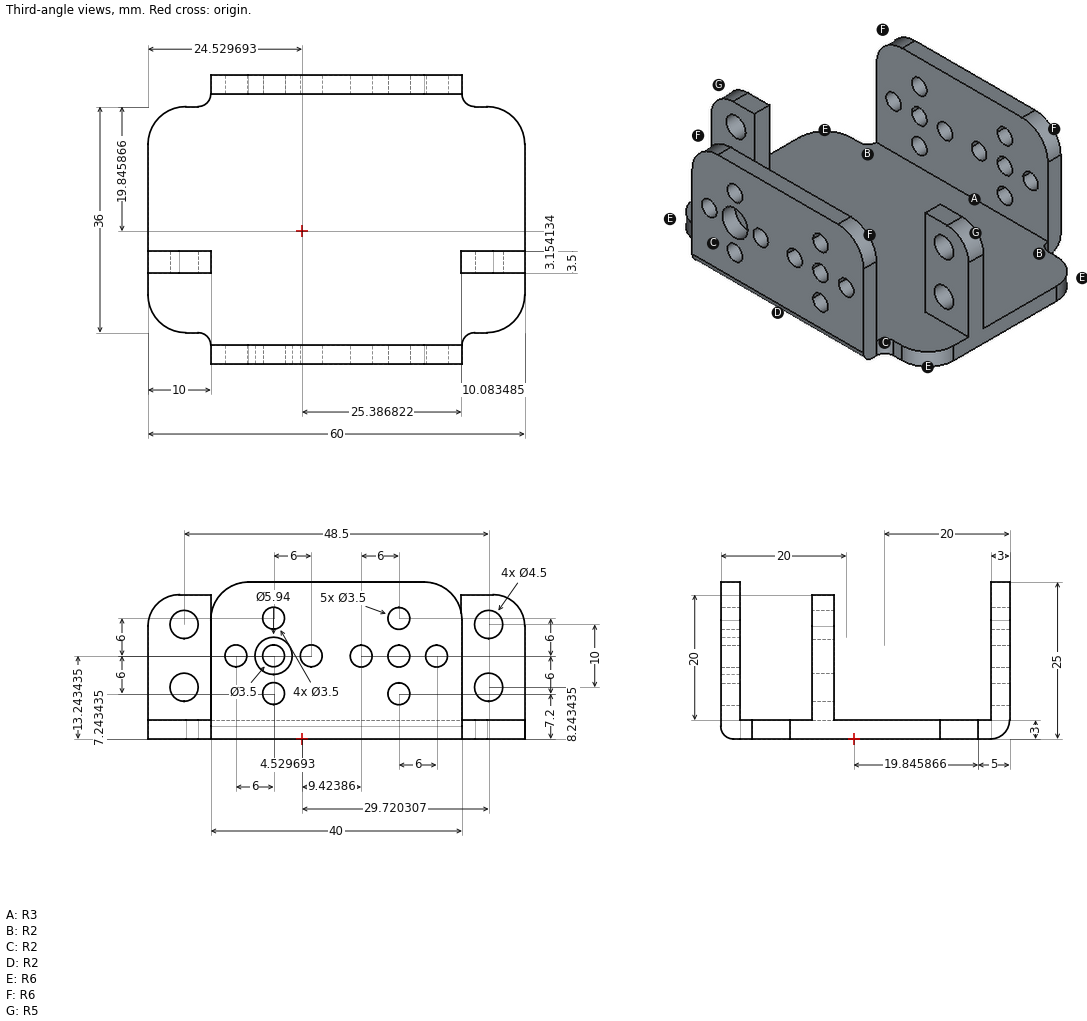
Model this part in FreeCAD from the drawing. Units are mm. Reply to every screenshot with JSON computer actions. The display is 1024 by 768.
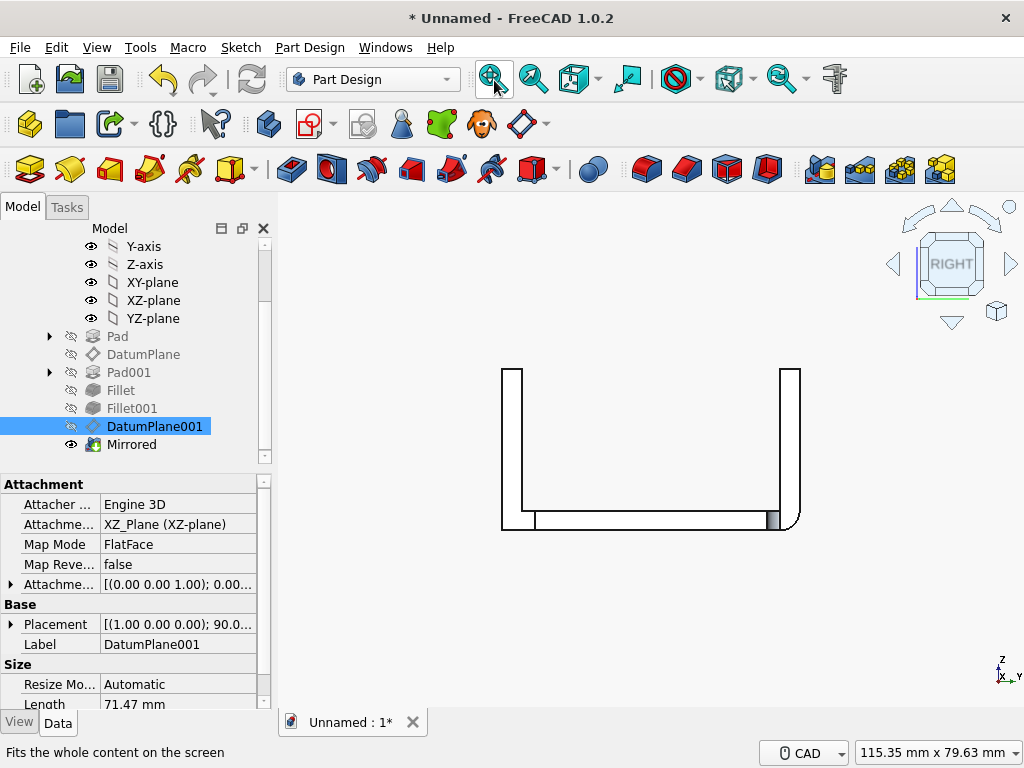
{"action": "key", "text": "5"}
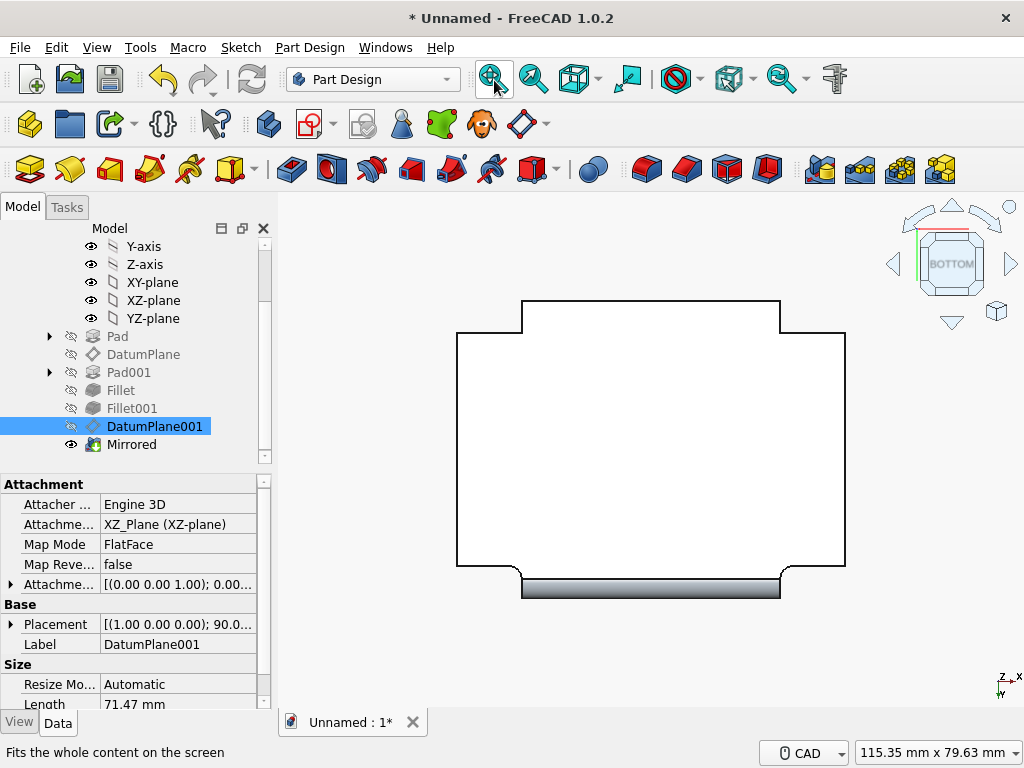
{"action": "scroll", "coordinate": [780, 332], "scroll_direction": "up", "scroll_amount": 4}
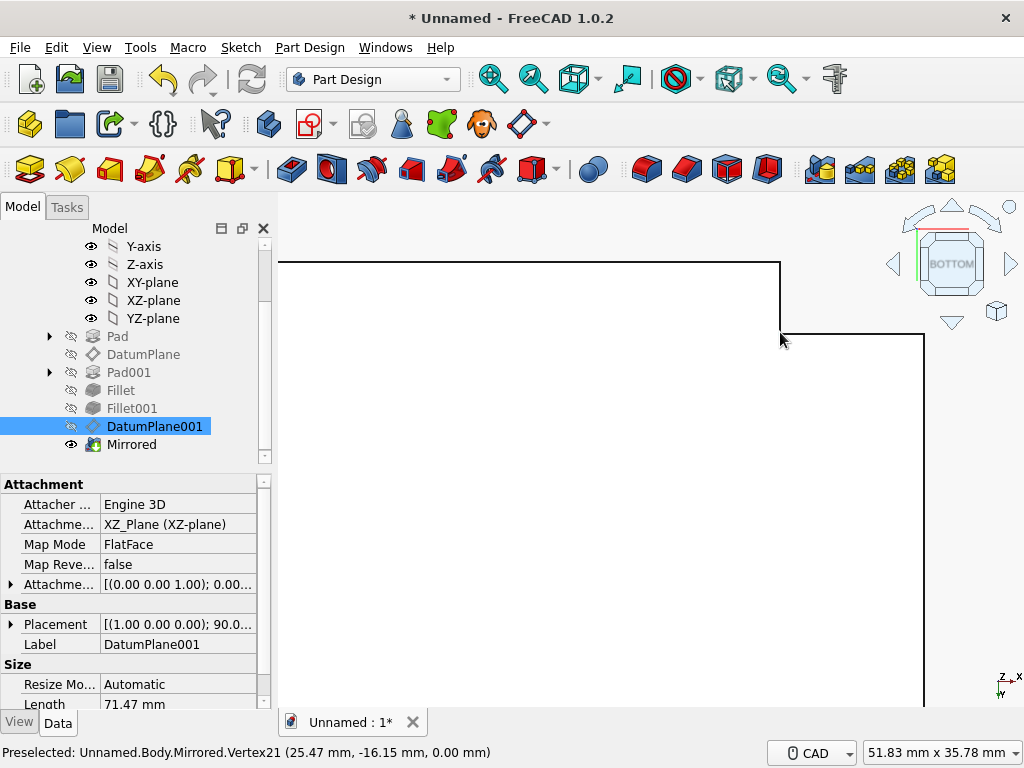
{"action": "left_click", "coordinate": [494, 80]}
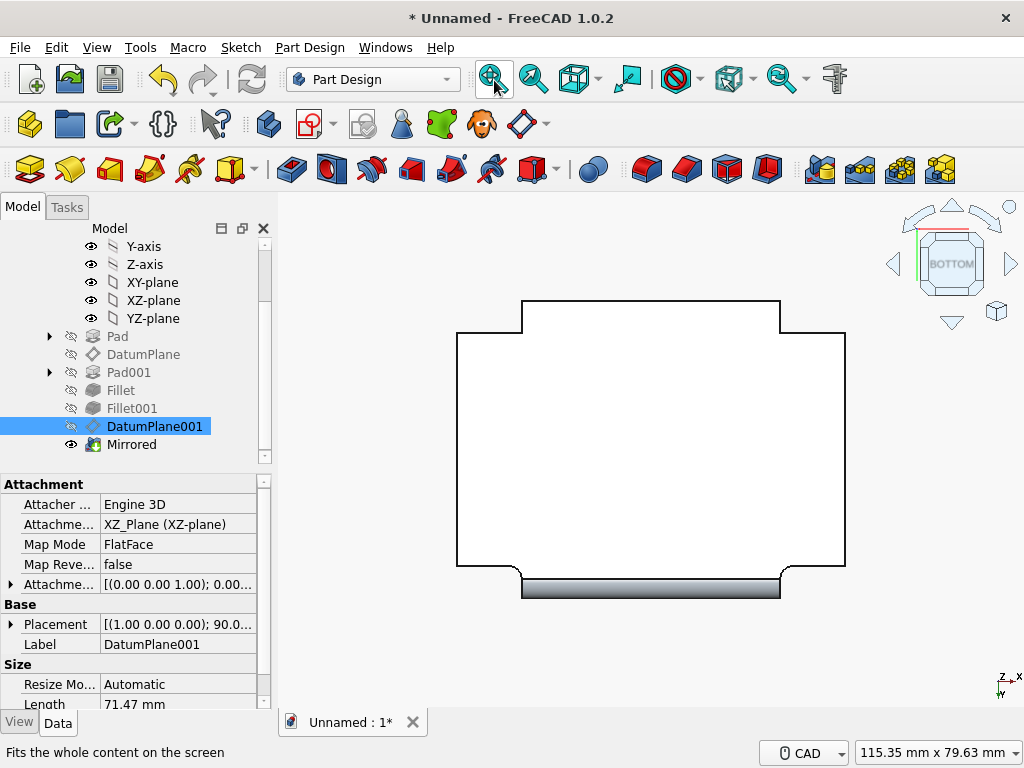
{"action": "key", "text": "4"}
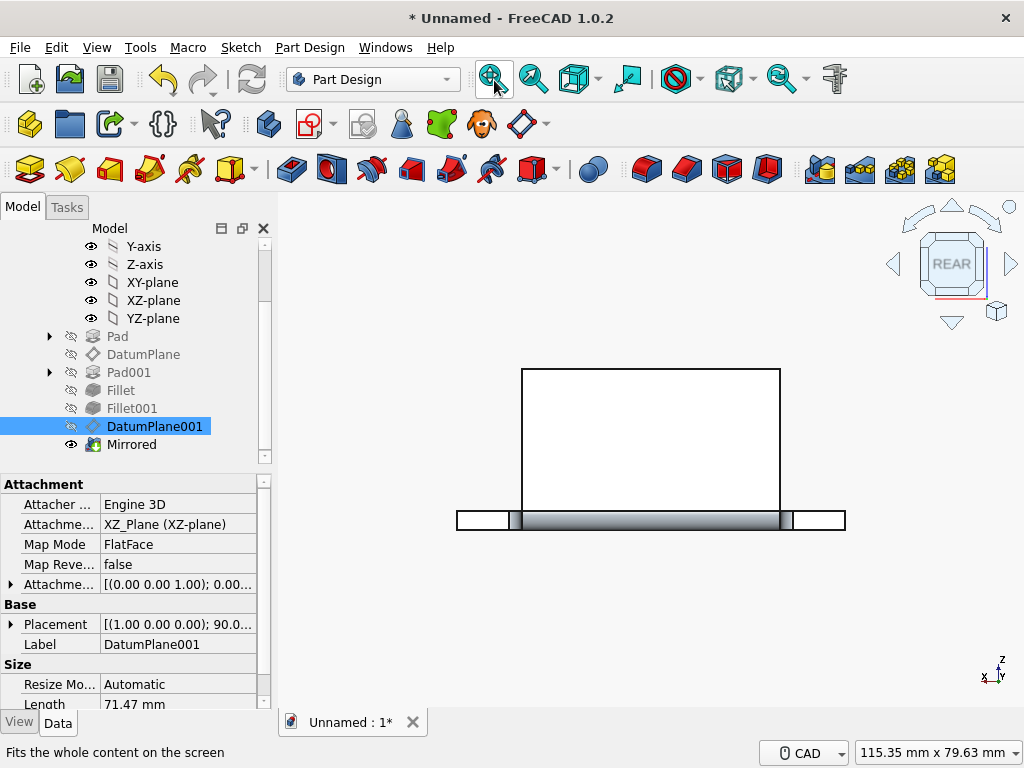
{"action": "scroll", "coordinate": [522, 520], "scroll_direction": "up", "scroll_amount": 4}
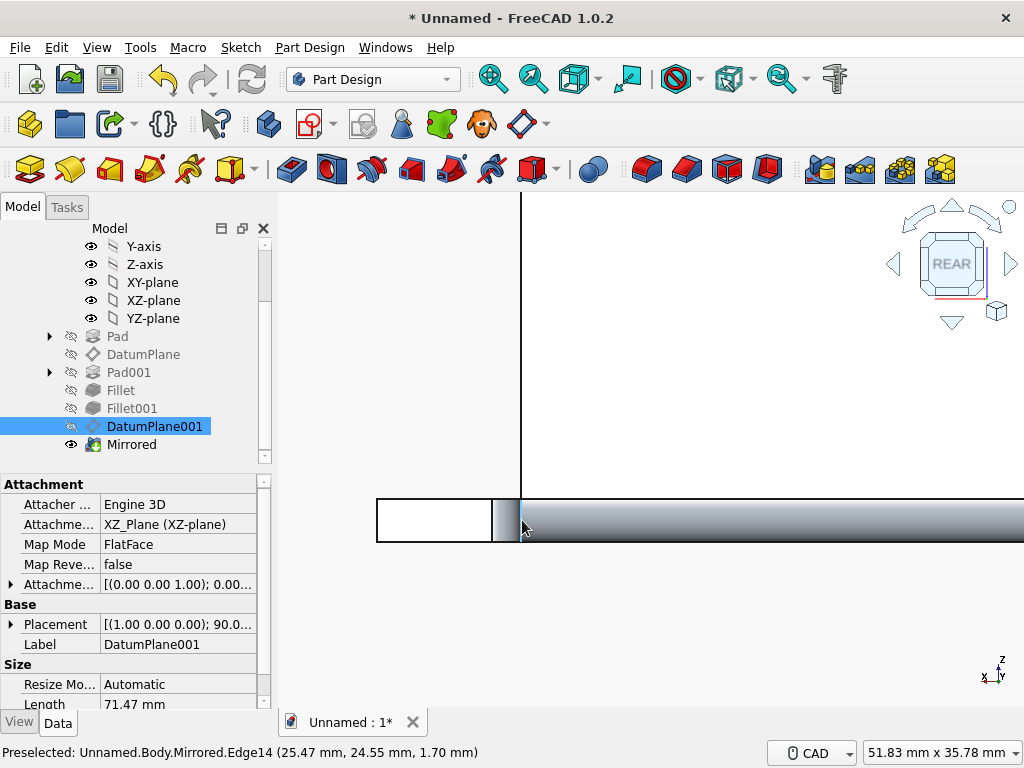
{"action": "left_click", "coordinate": [494, 80]}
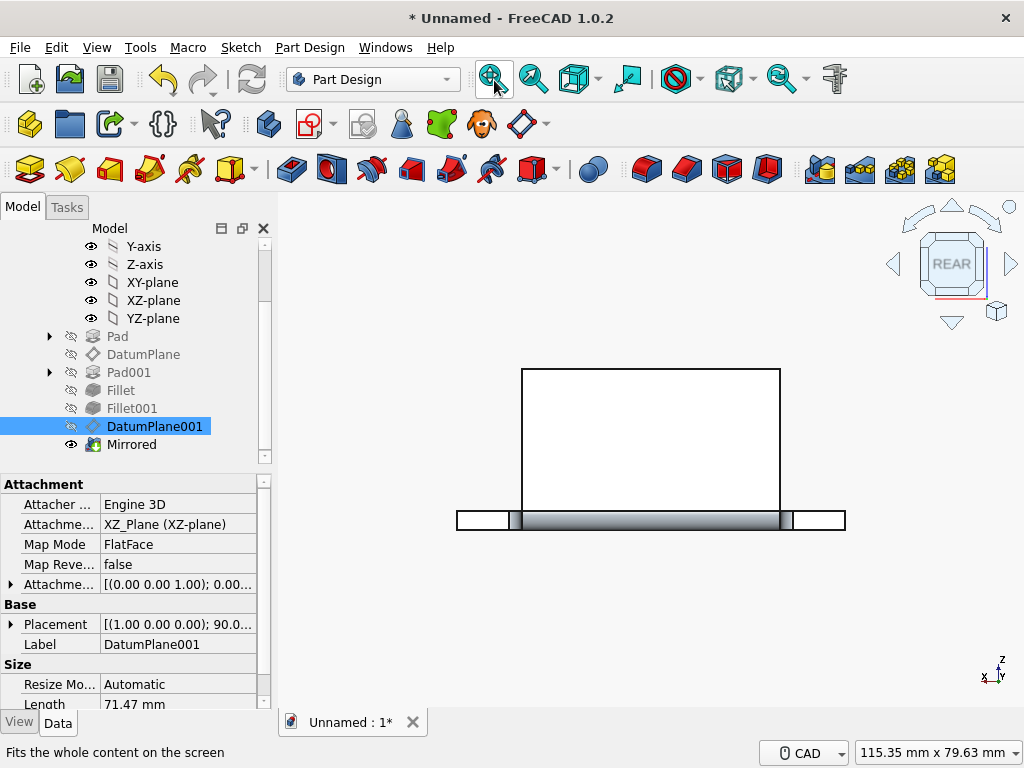
{"action": "key", "text": "6"}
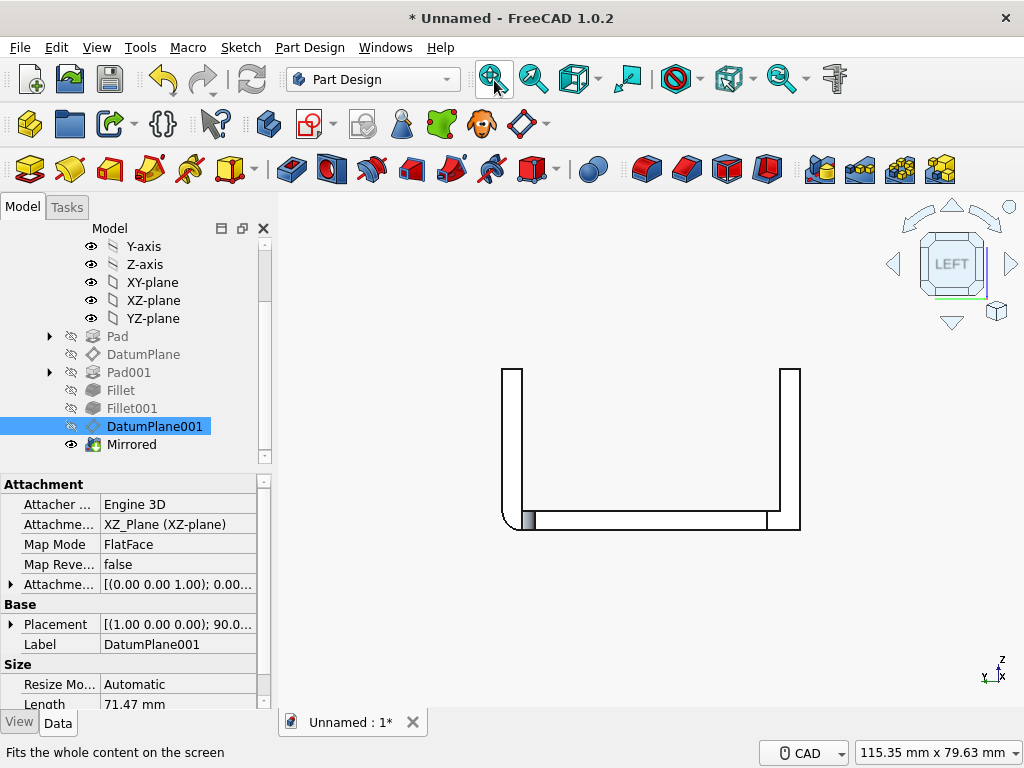
{"action": "left_click", "coordinate": [494, 80]}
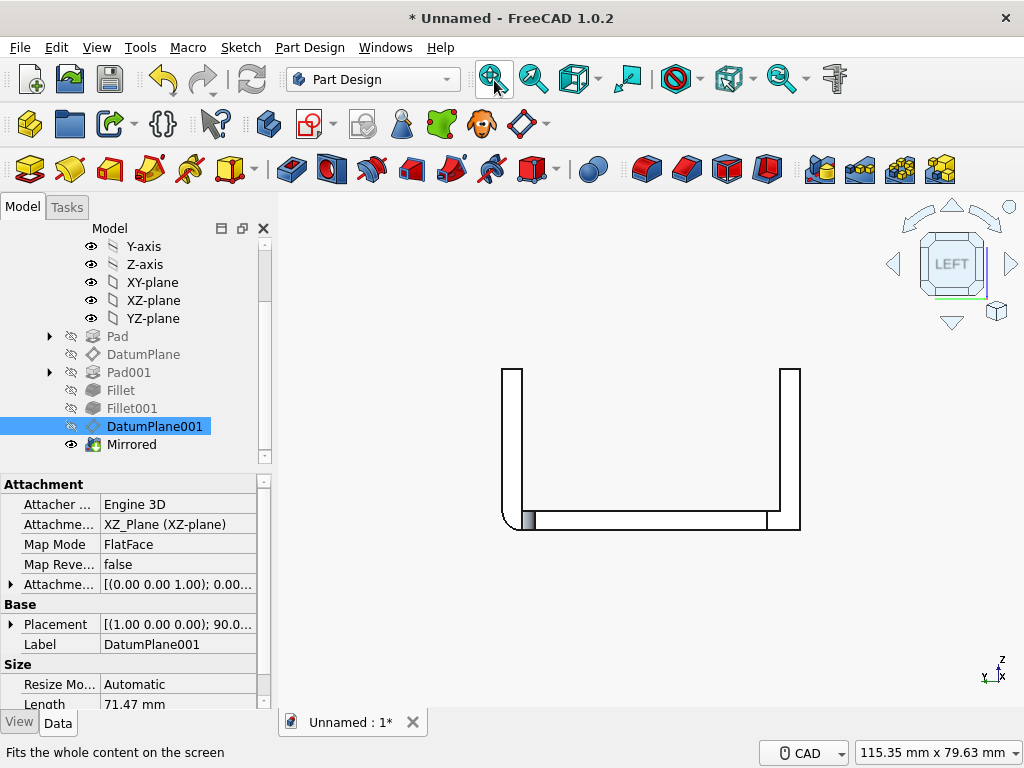
{"action": "scroll", "coordinate": [767, 520], "scroll_direction": "up", "scroll_amount": 4}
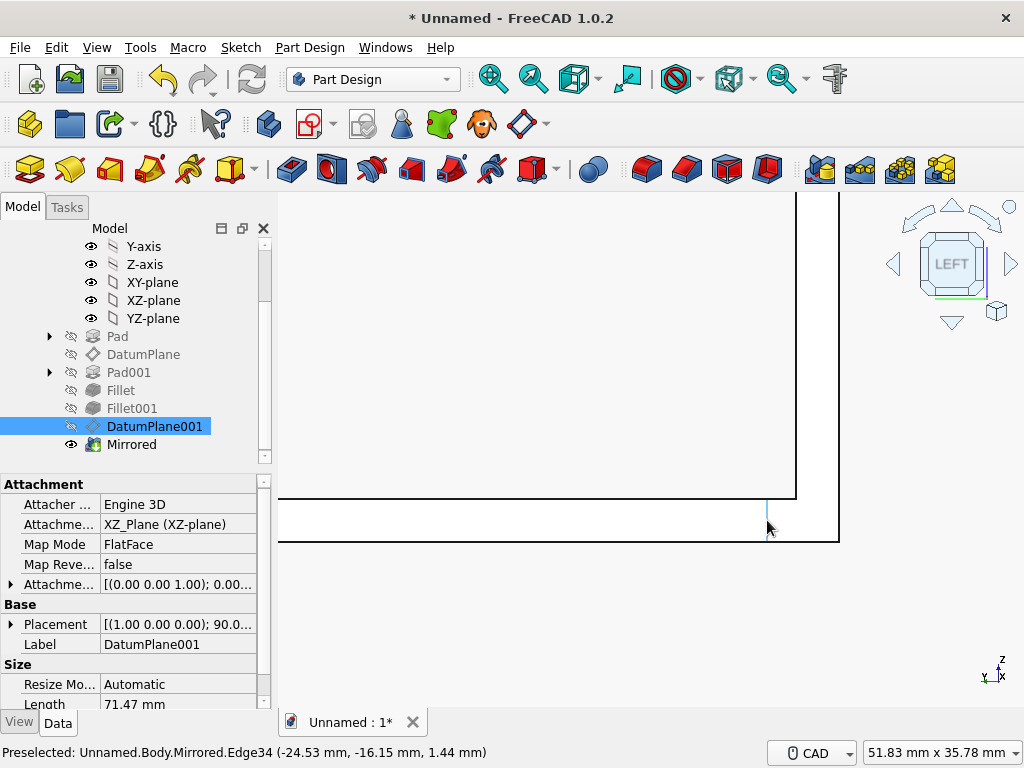
{"action": "left_click", "coordinate": [494, 80]}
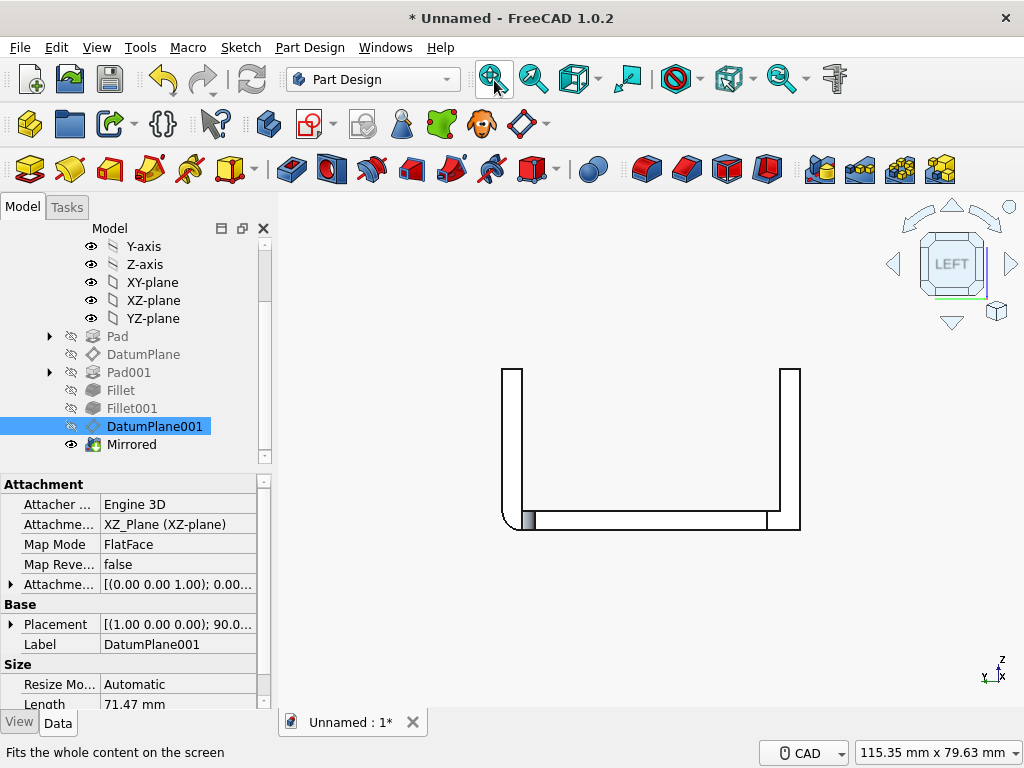
{"action": "key", "text": "v 3"}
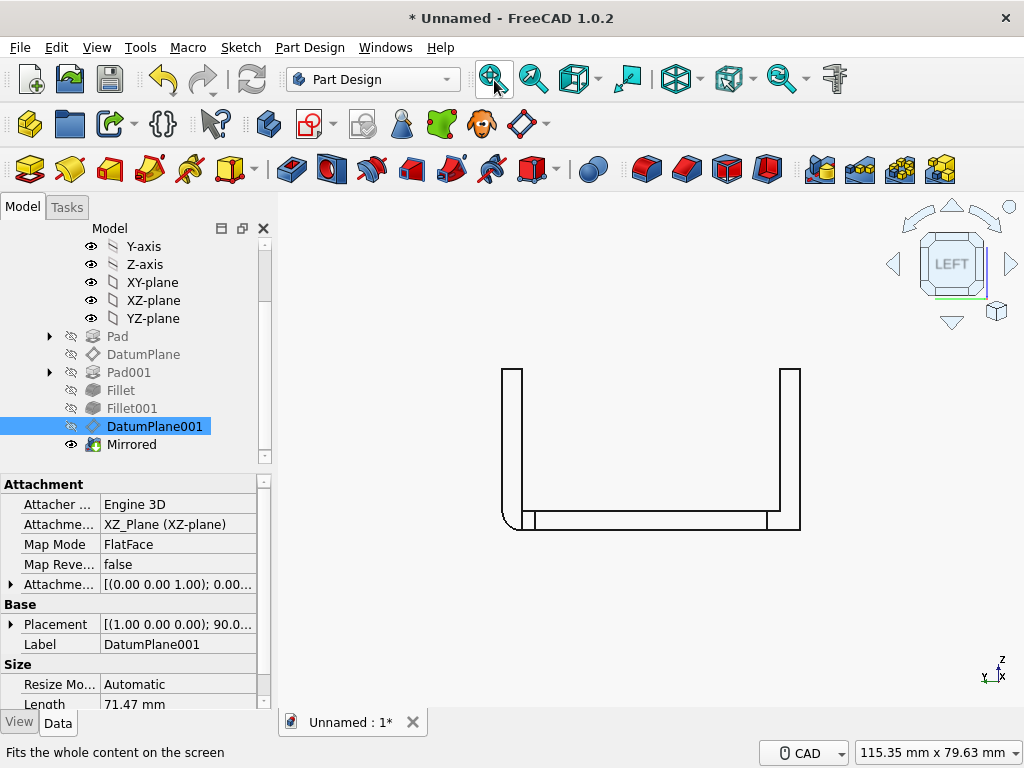
{"action": "key", "text": "0"}